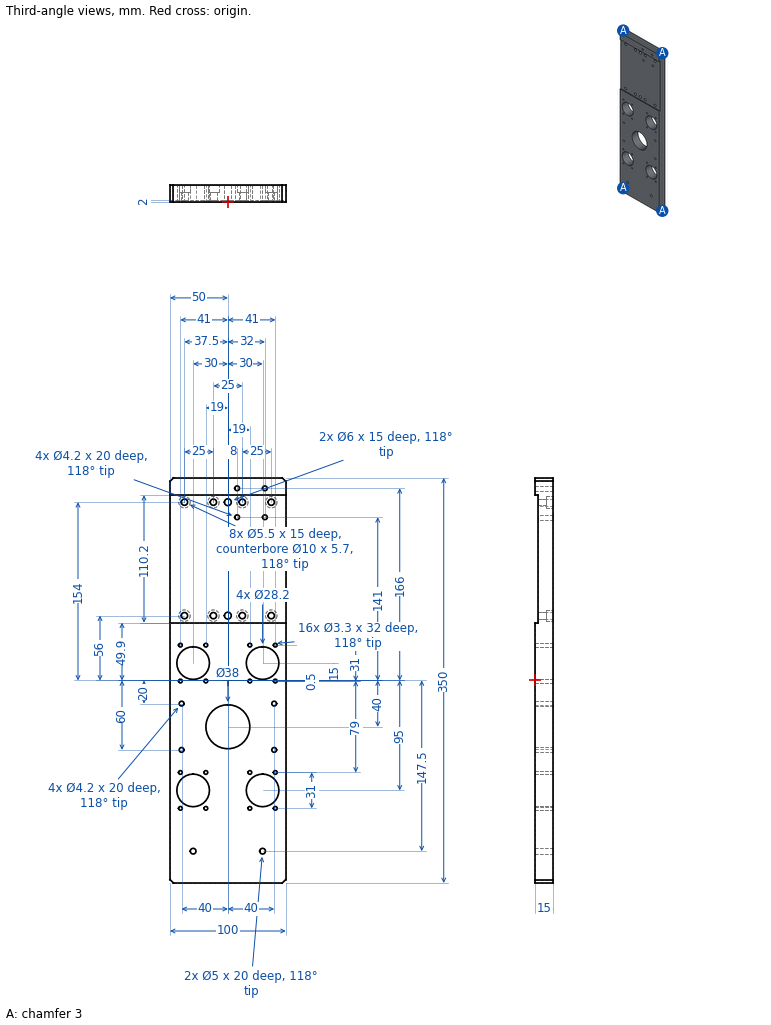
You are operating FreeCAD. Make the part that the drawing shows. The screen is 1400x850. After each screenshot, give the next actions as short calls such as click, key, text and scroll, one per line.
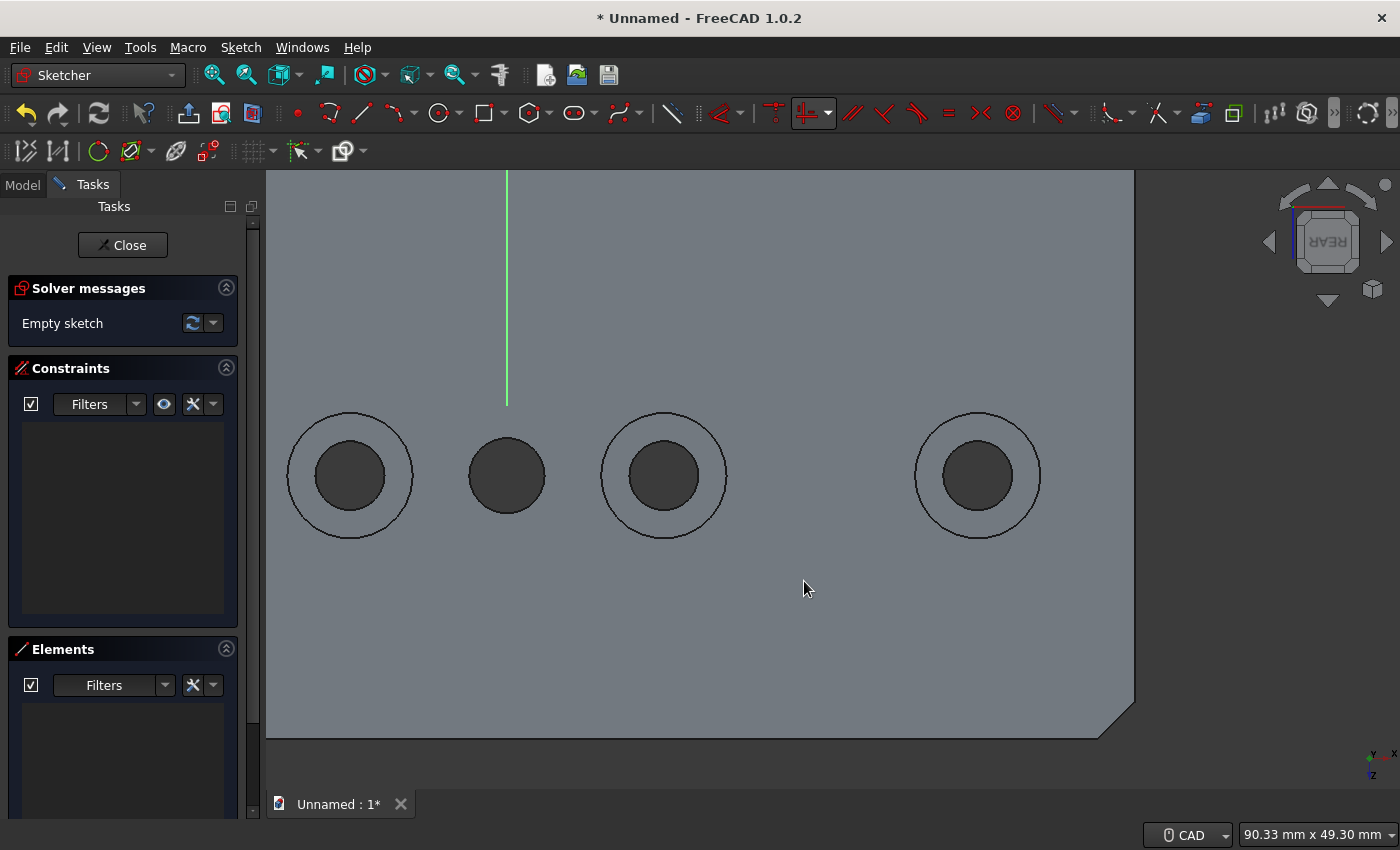
click(440, 114)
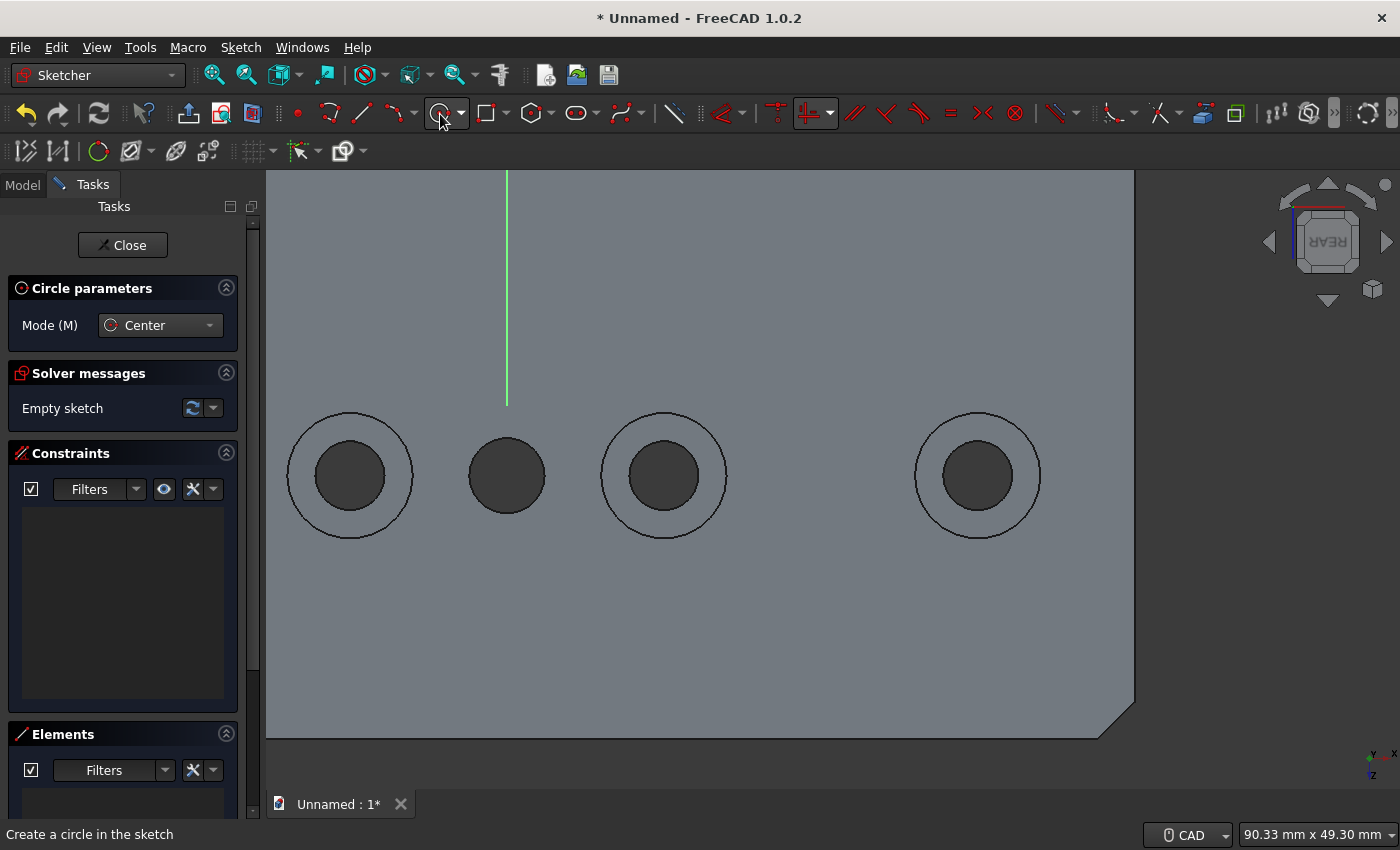
click(607, 313)
click(626, 294)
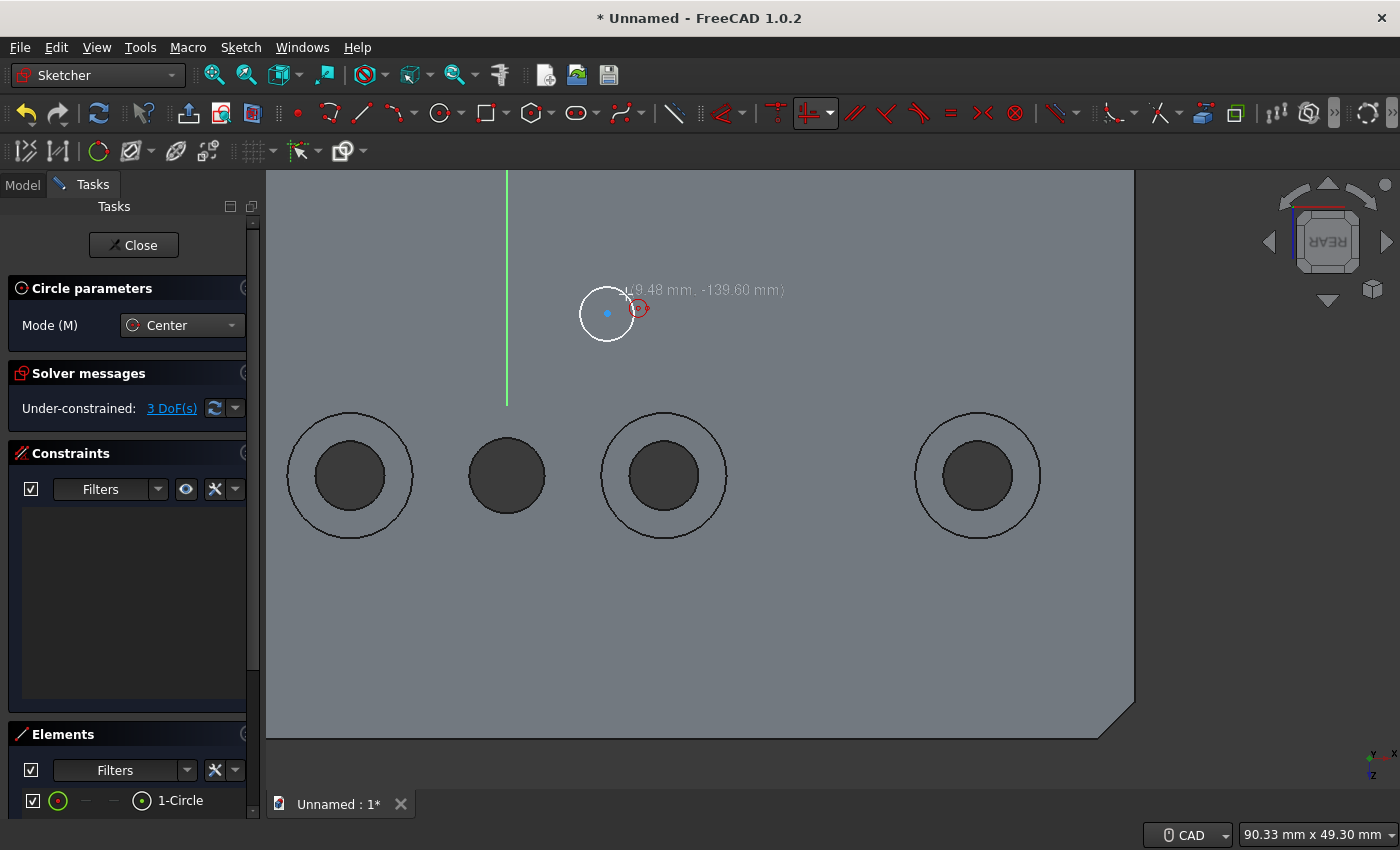
click(909, 313)
click(927, 294)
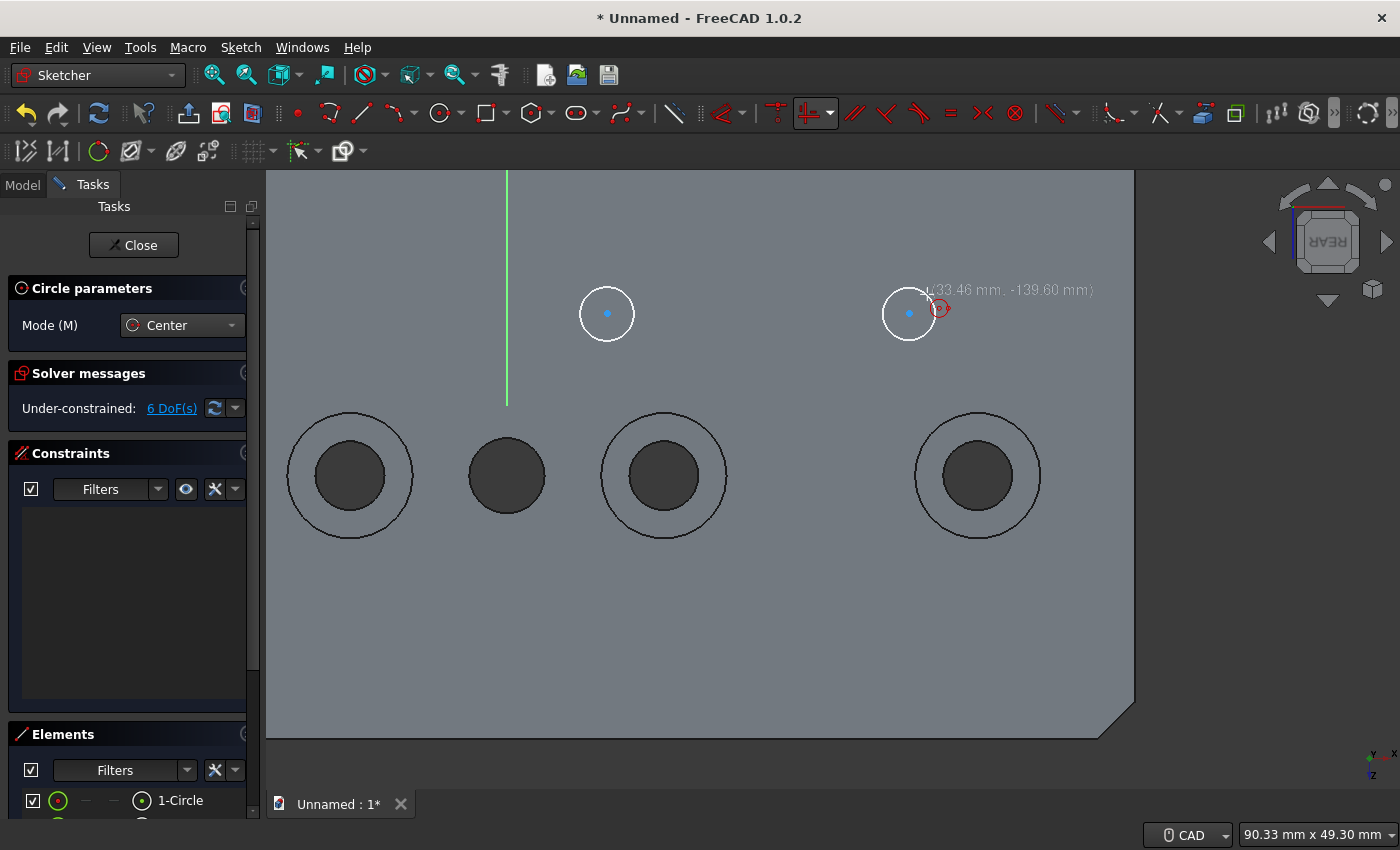
click(607, 626)
click(626, 608)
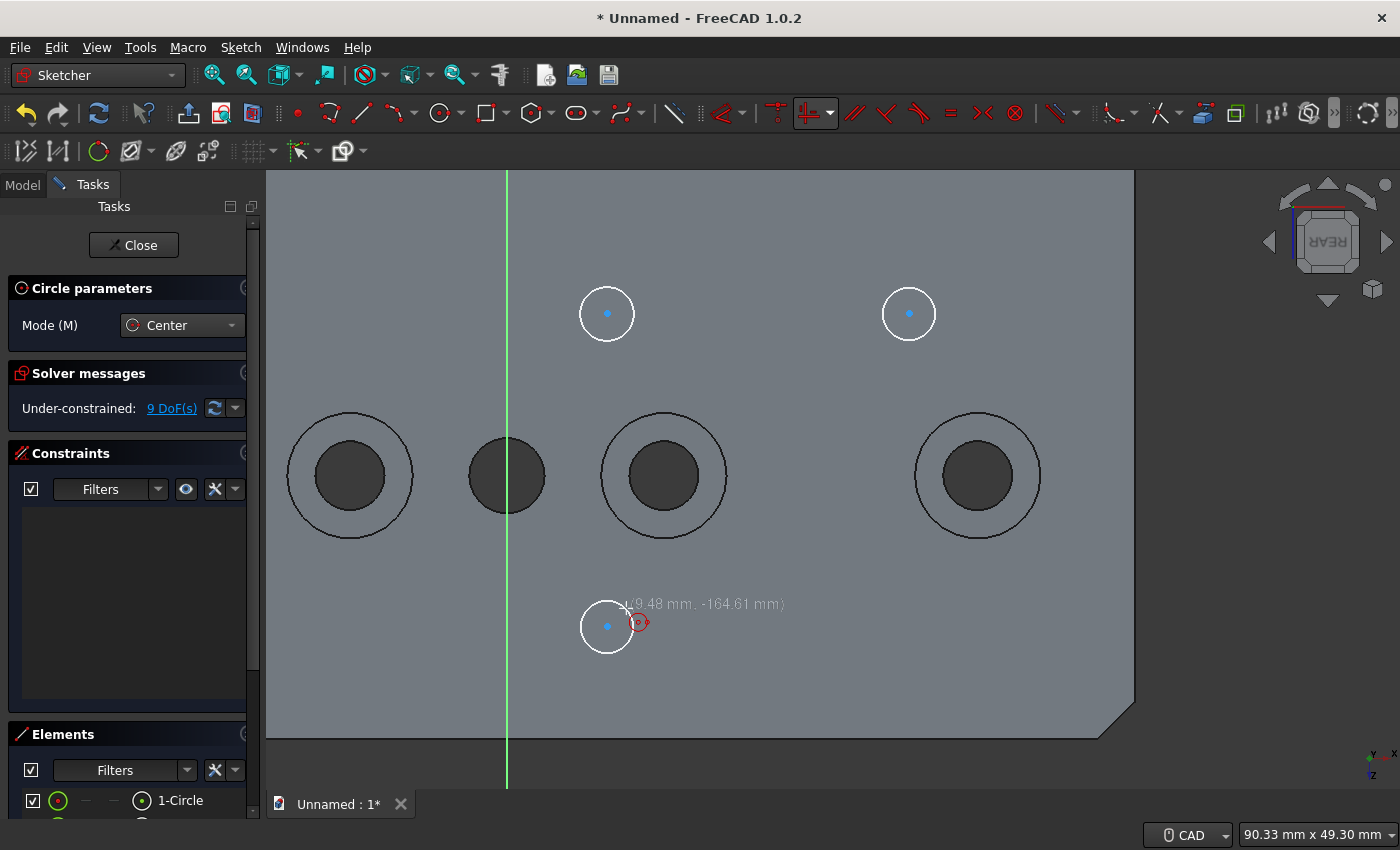
click(909, 626)
click(927, 608)
key(Escape)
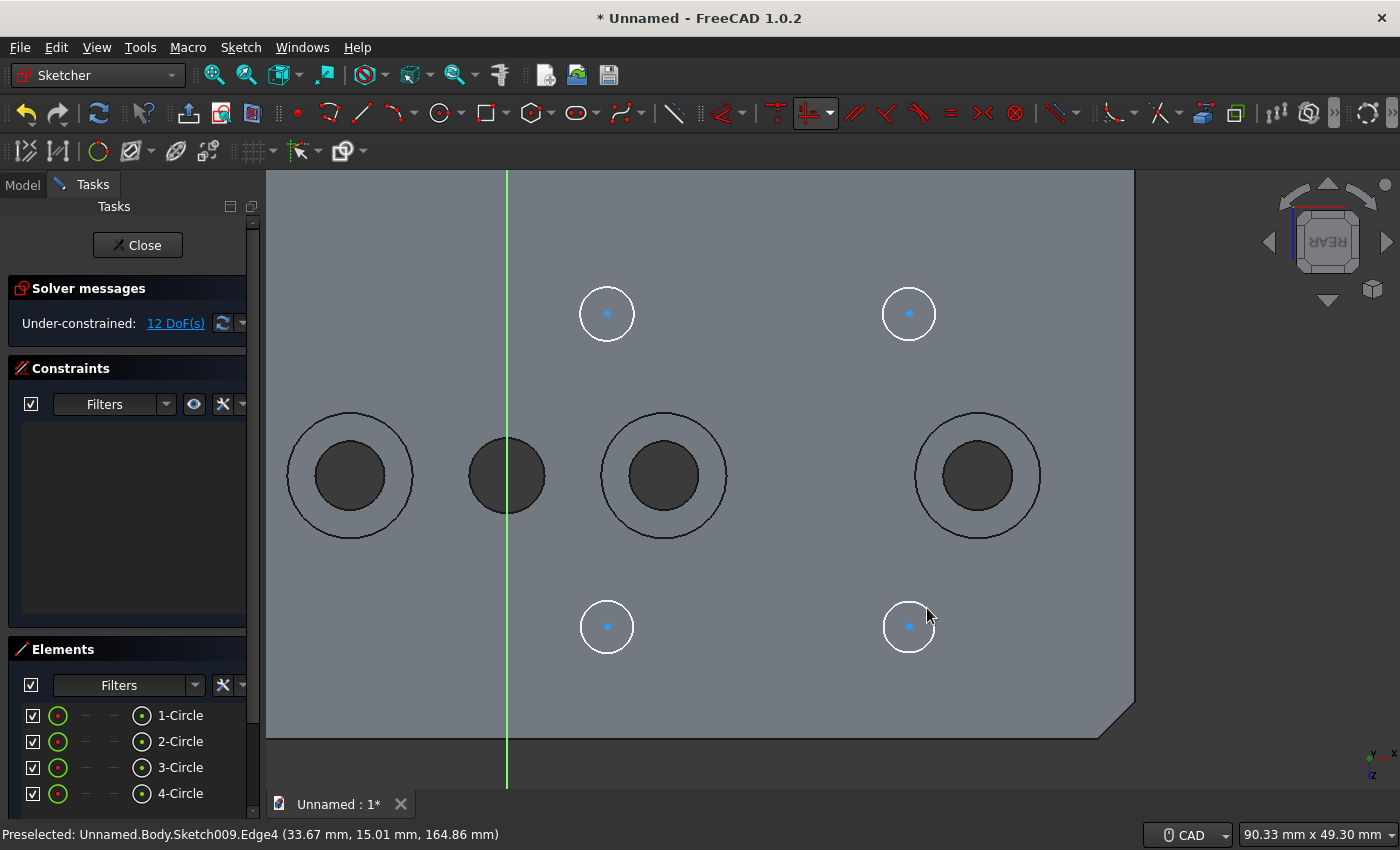
click(626, 295)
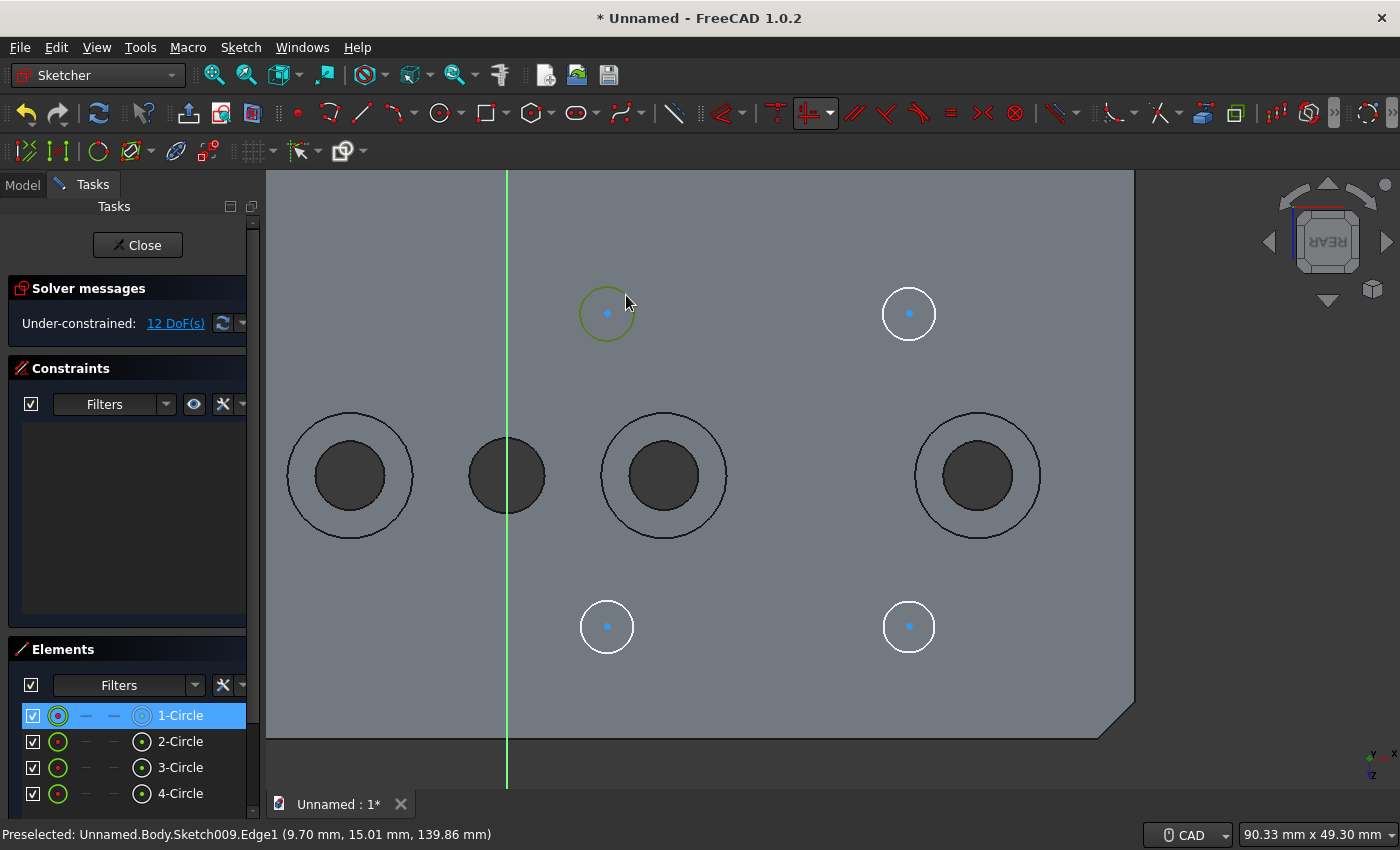
click(927, 295)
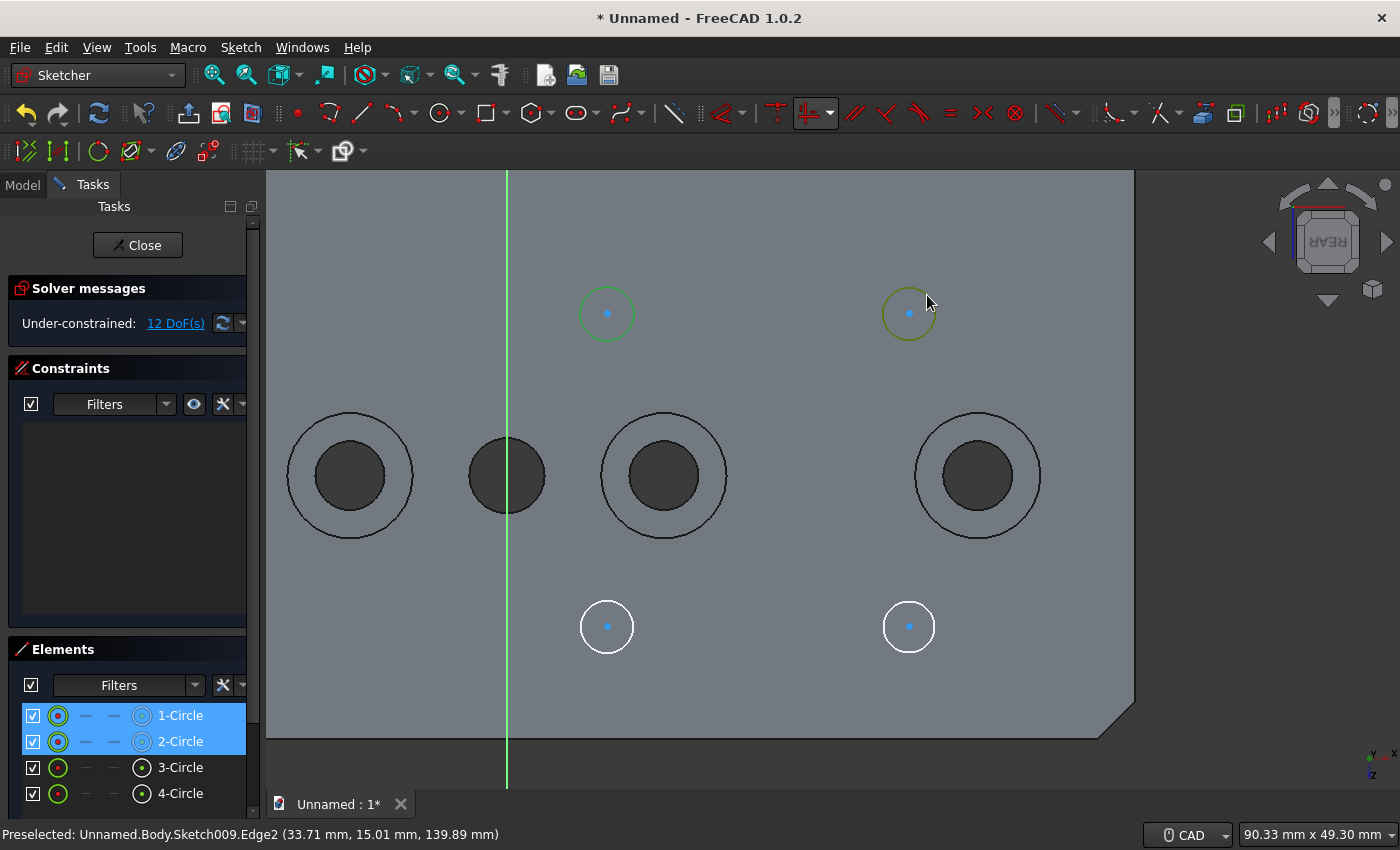
click(625, 608)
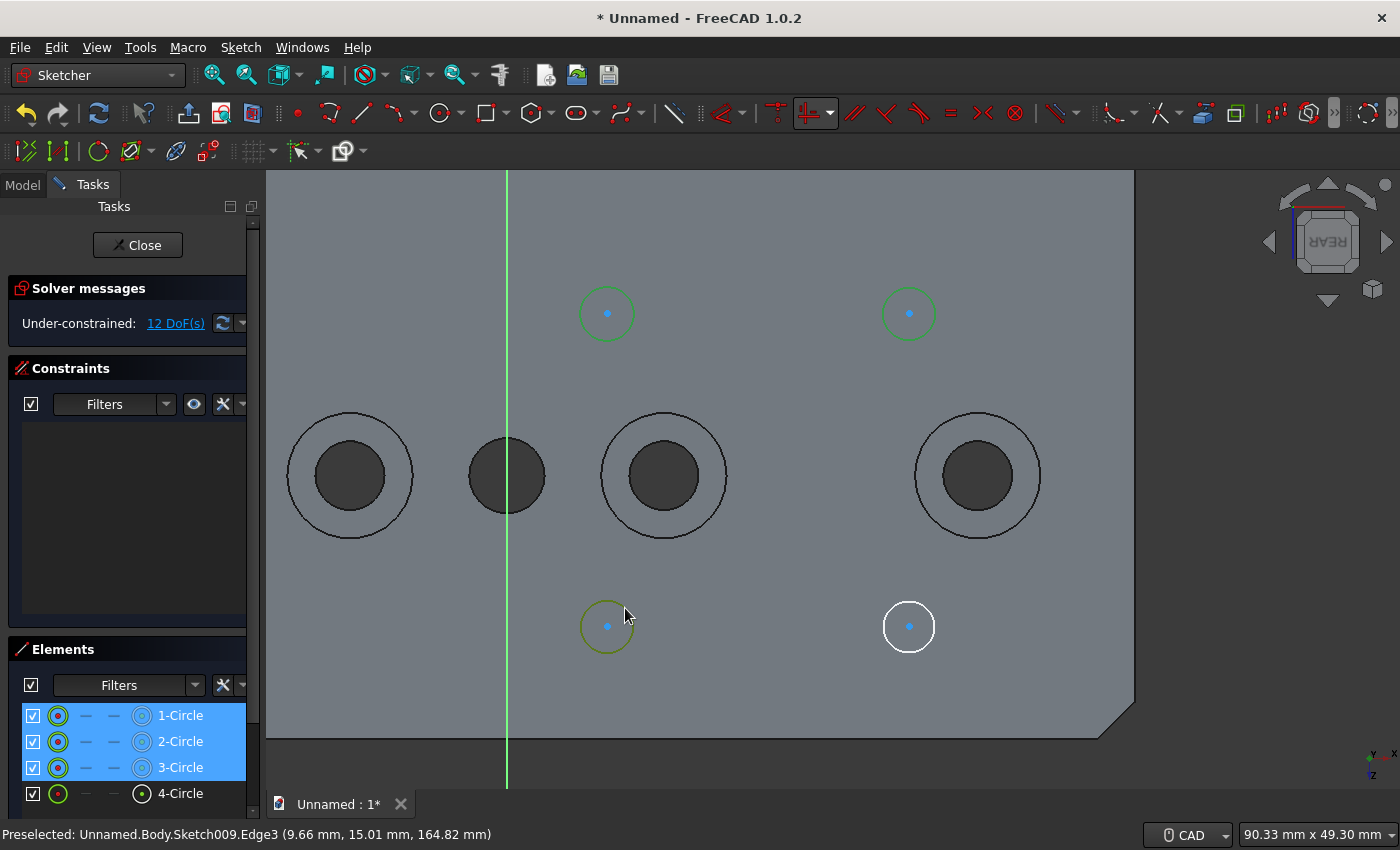
click(927, 609)